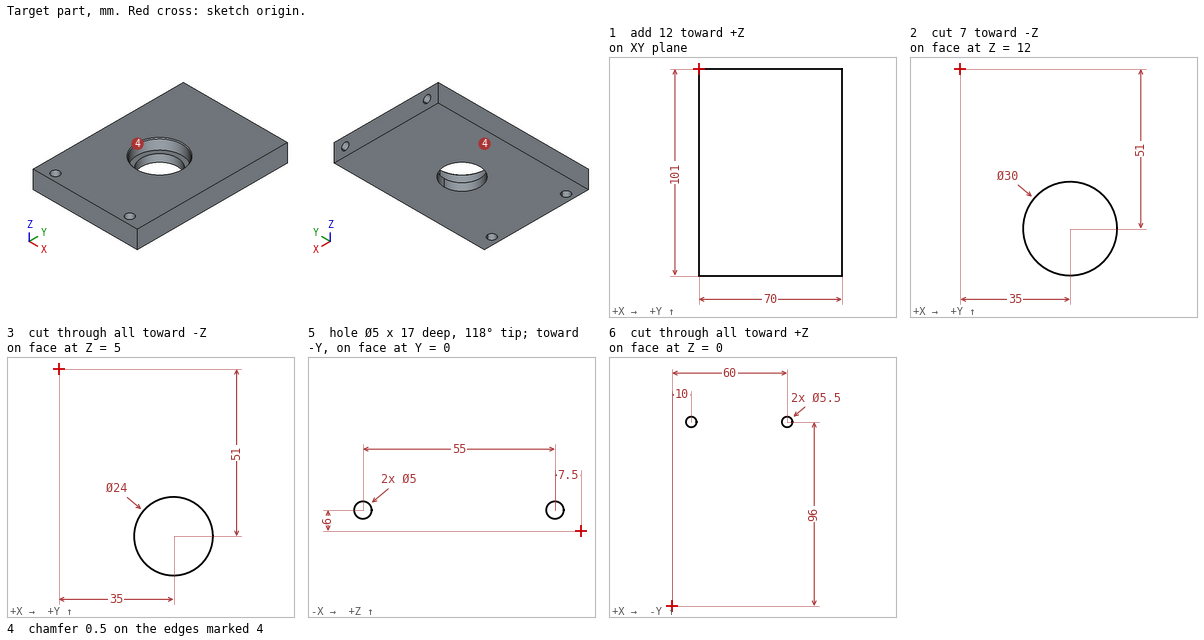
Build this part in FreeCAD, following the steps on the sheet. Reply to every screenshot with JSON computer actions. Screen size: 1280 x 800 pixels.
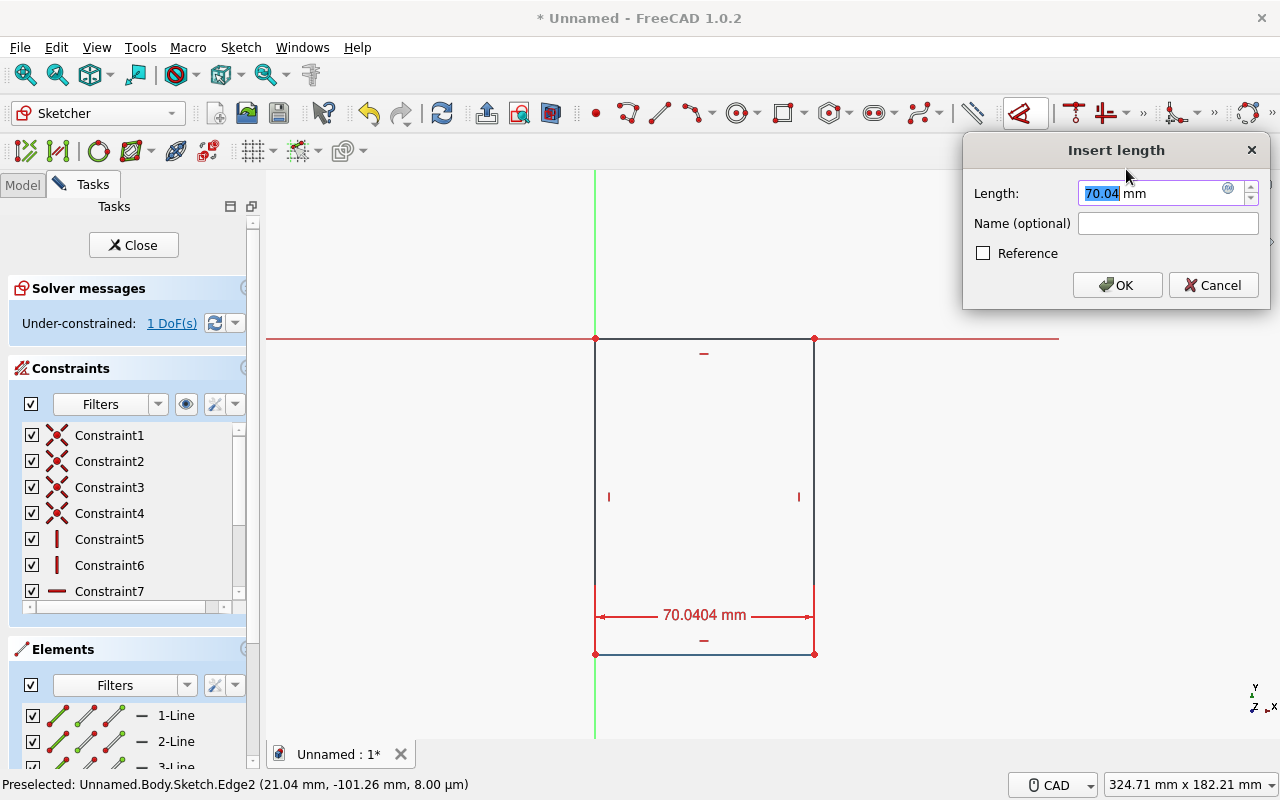
{"action": "type", "text": "70"}
{"action": "key", "text": "Return"}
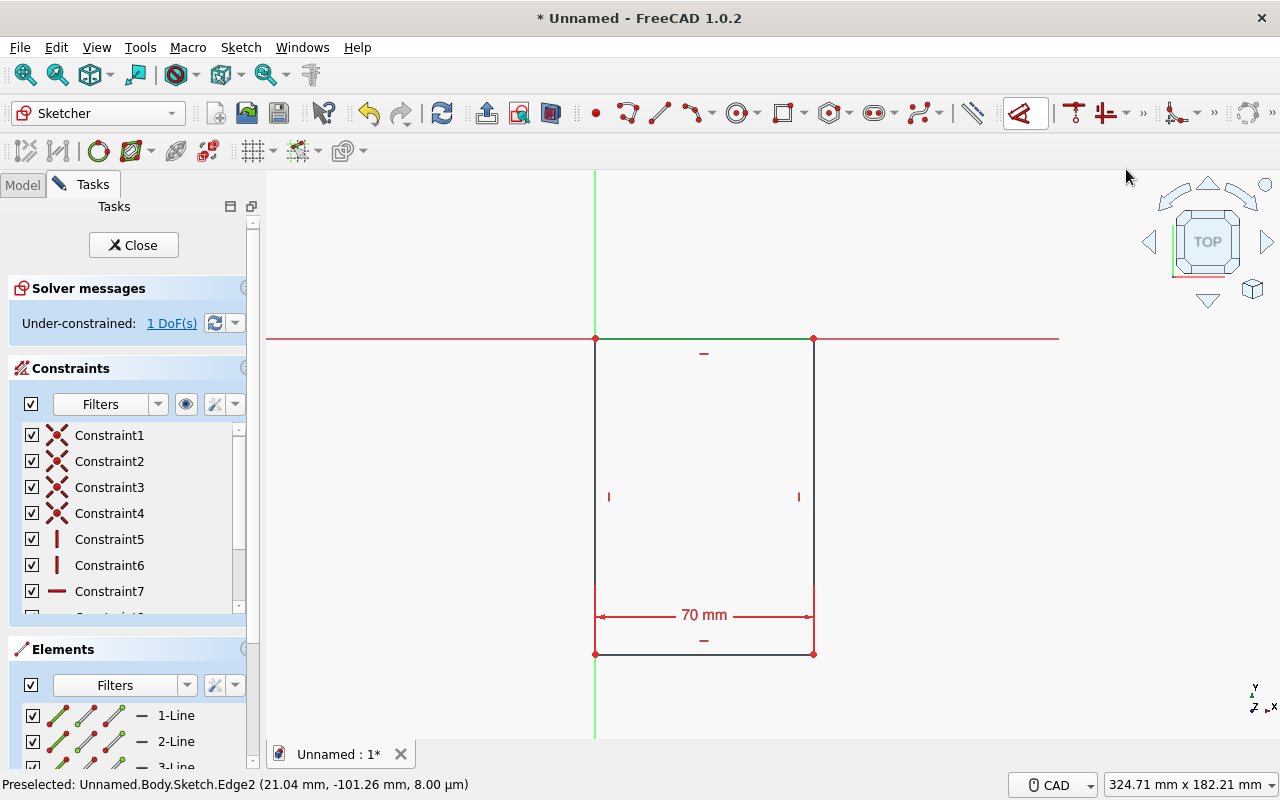
{"action": "left_click", "coordinate": [595, 434]}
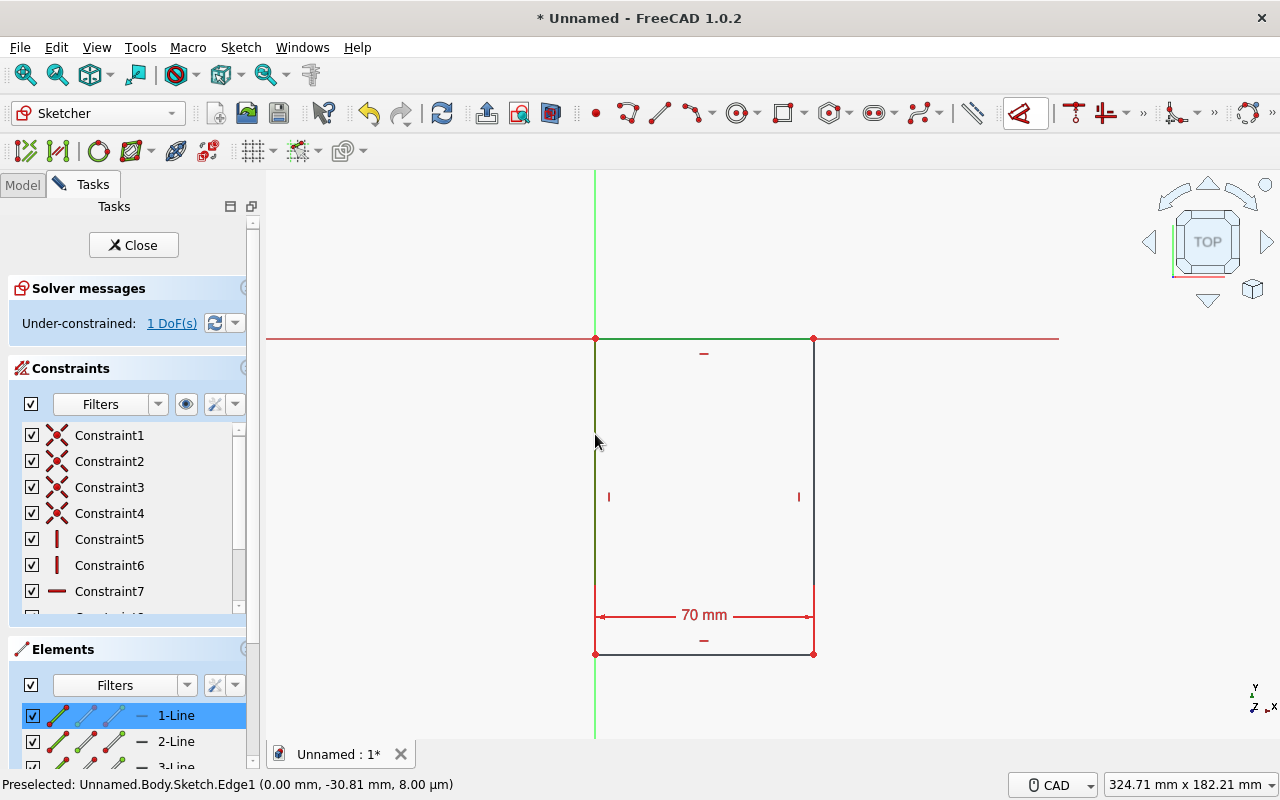
{"action": "key", "text": "i"}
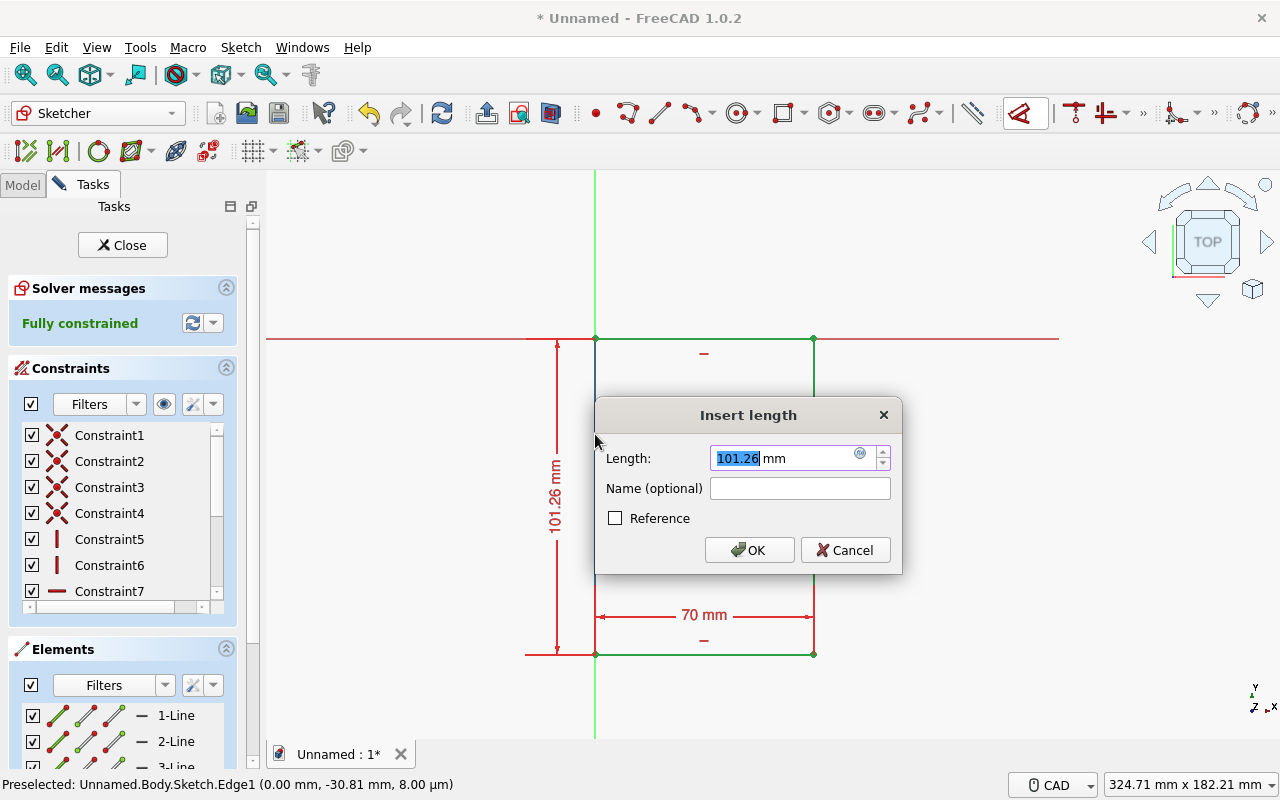
{"action": "type", "text": "101"}
{"action": "key", "text": "Return"}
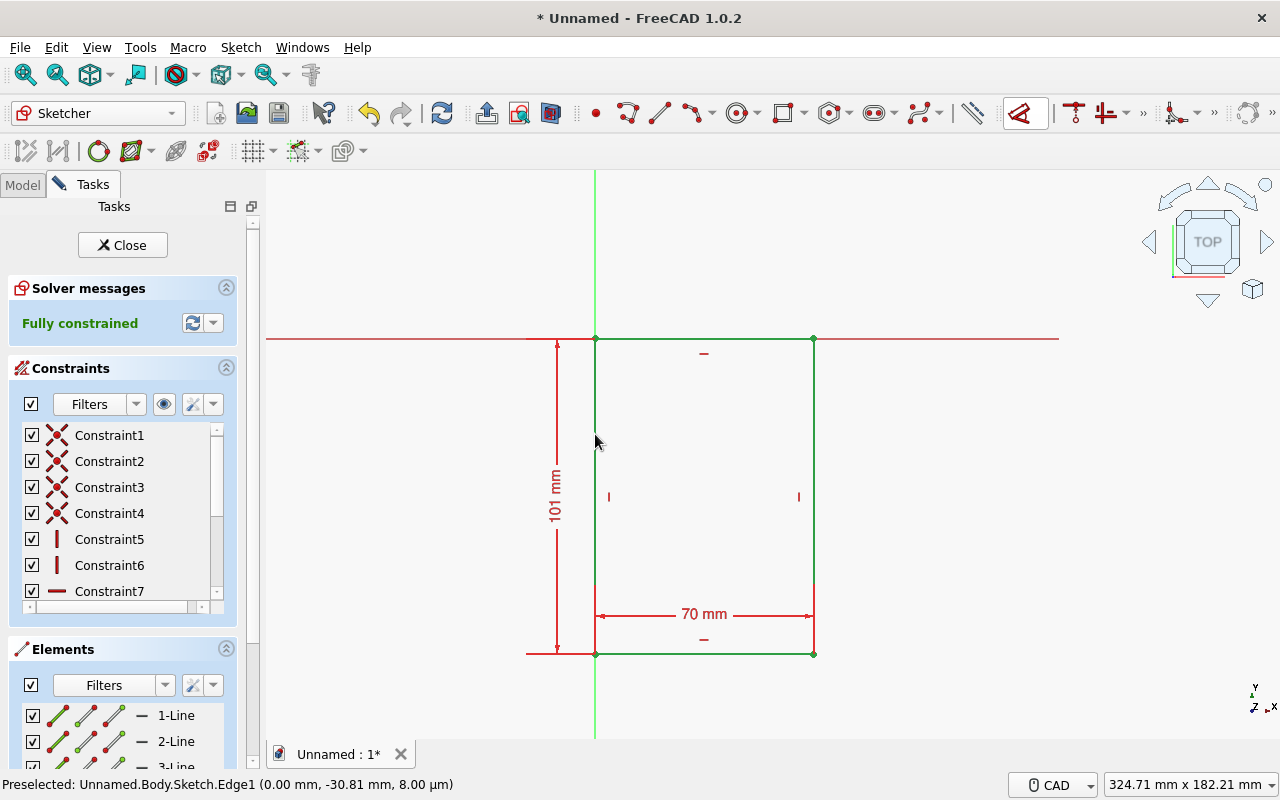
{"action": "left_click", "coordinate": [123, 245]}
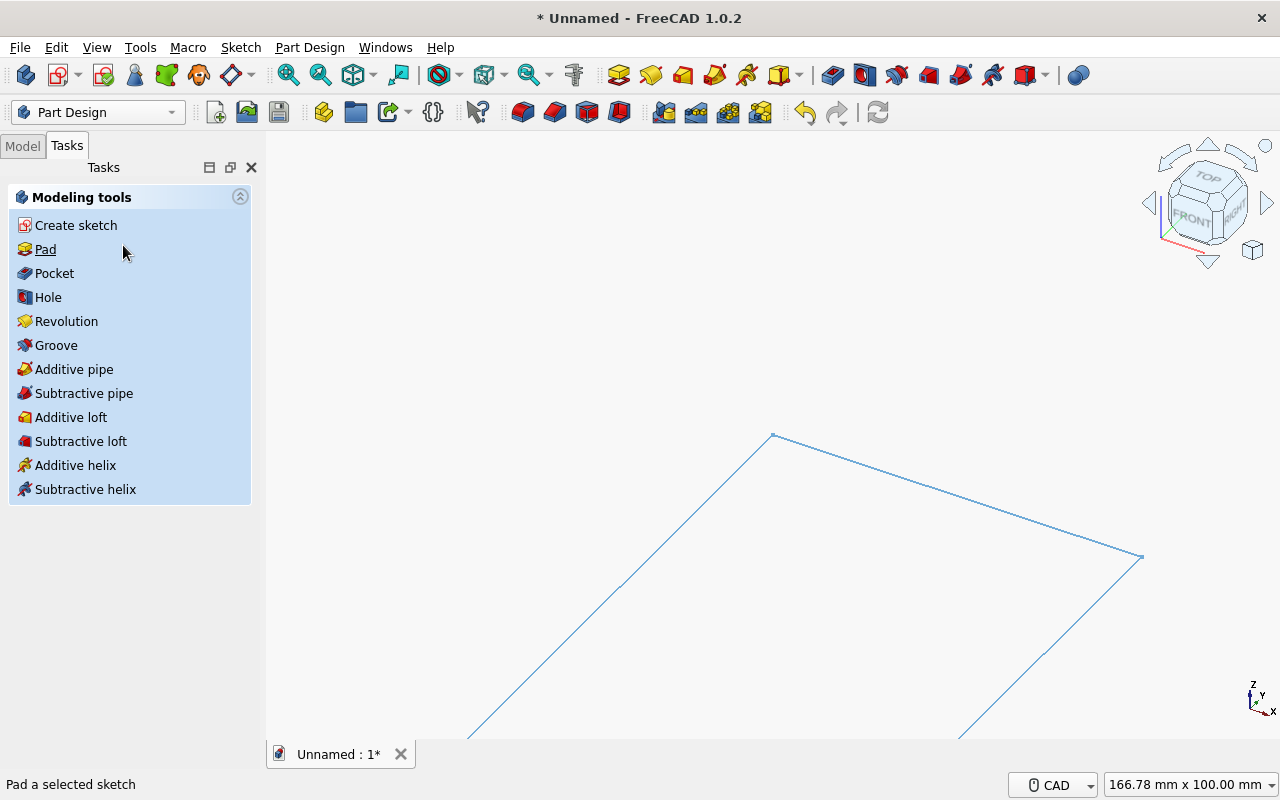
{"action": "left_click", "coordinate": [620, 76]}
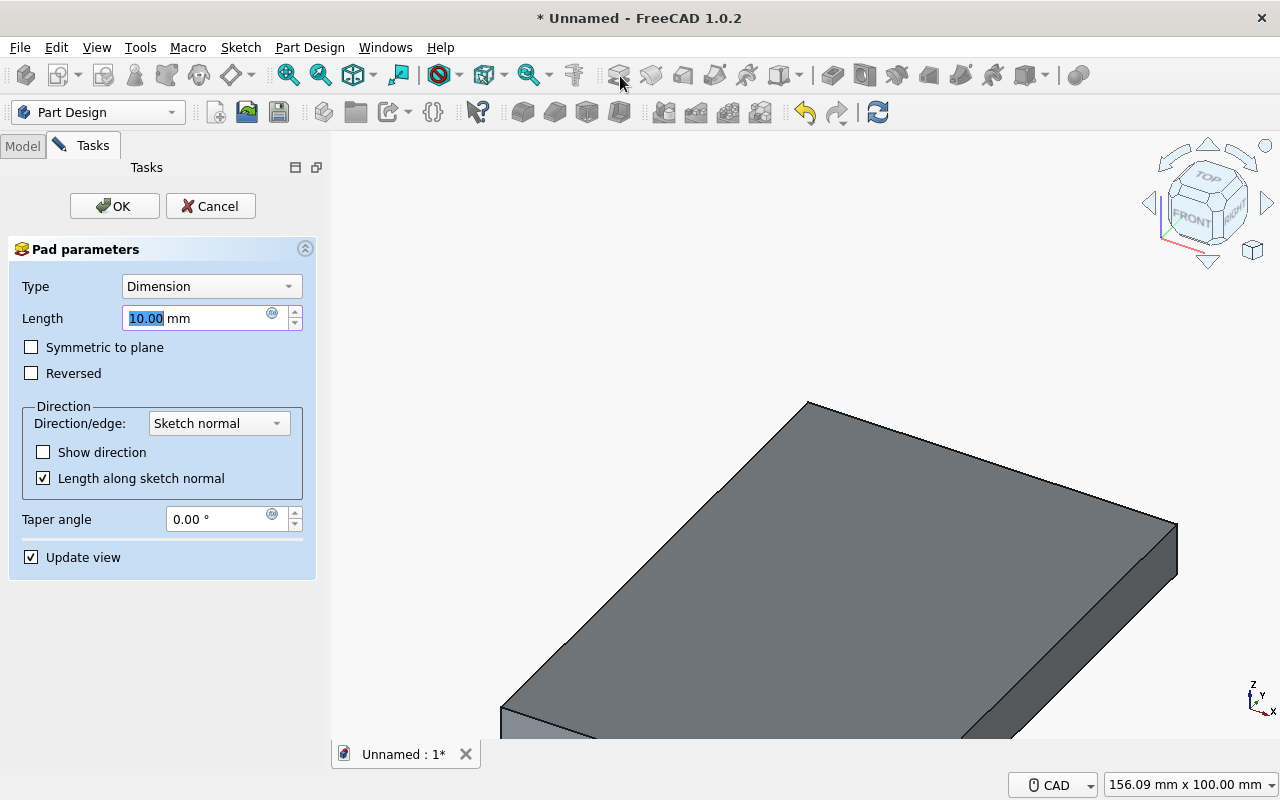
{"action": "type", "text": "12"}
{"action": "key", "text": "Tab"}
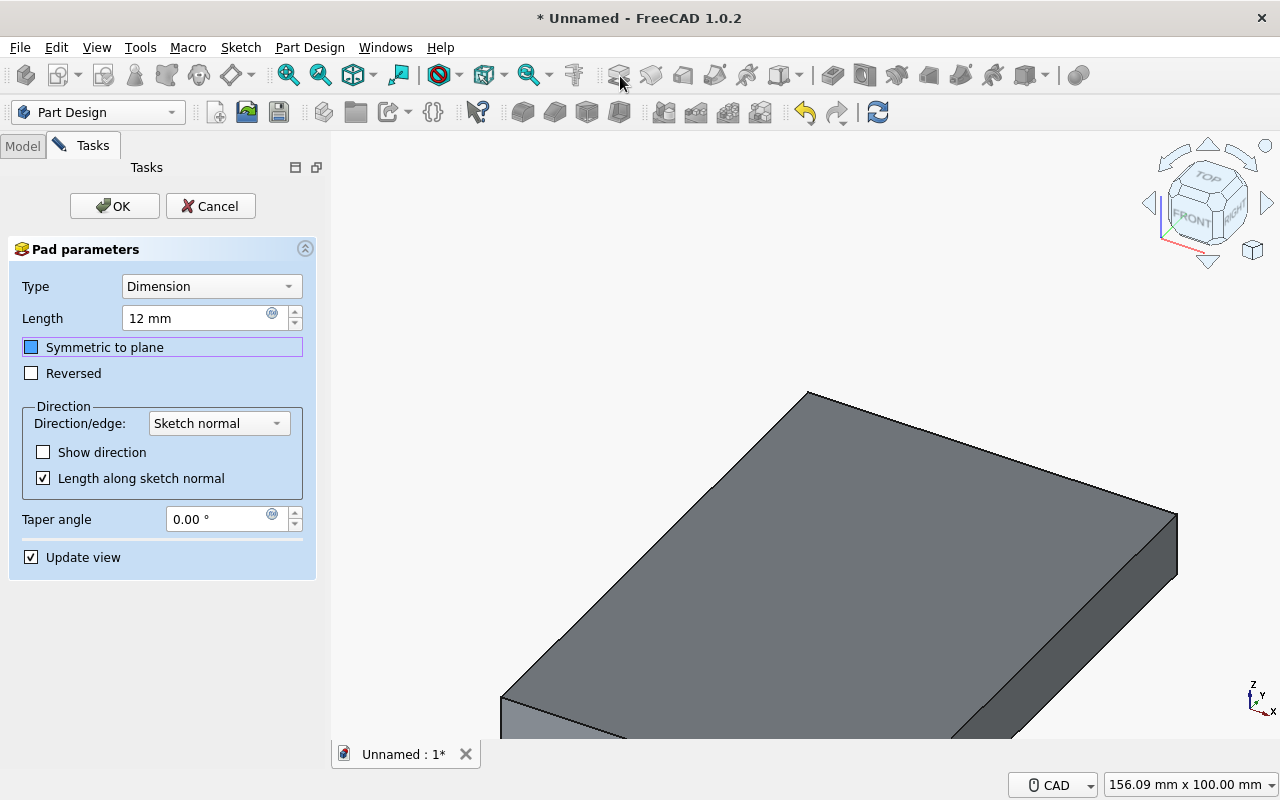
{"action": "left_click", "coordinate": [115, 206]}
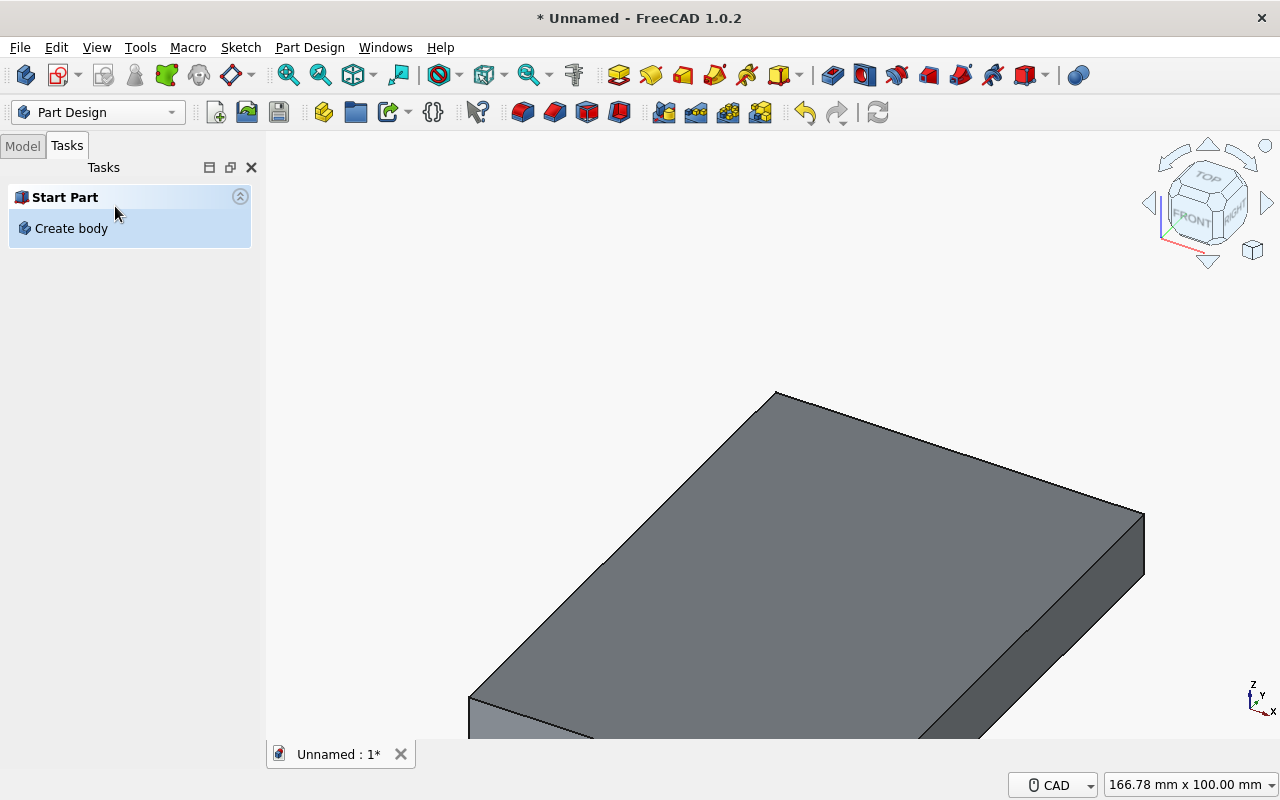
{"action": "left_click", "coordinate": [290, 76]}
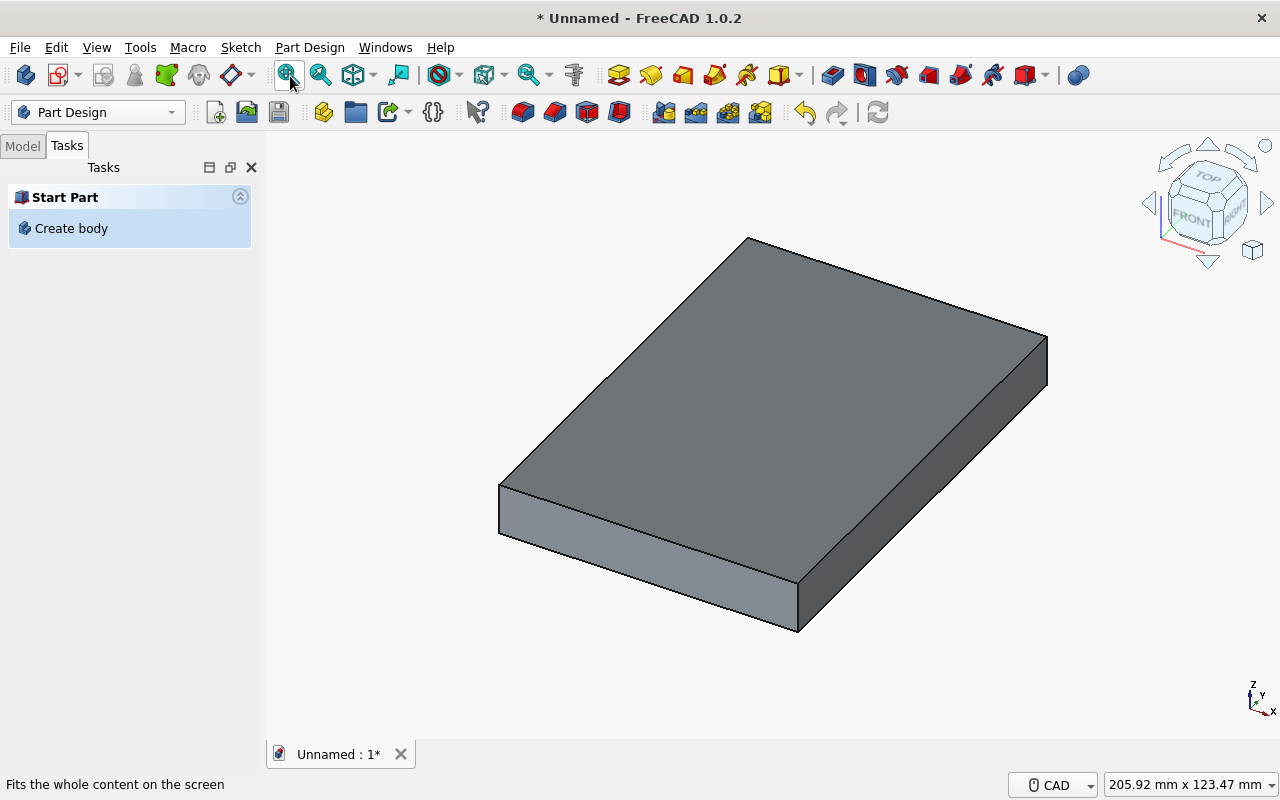
{"action": "left_click", "coordinate": [809, 375]}